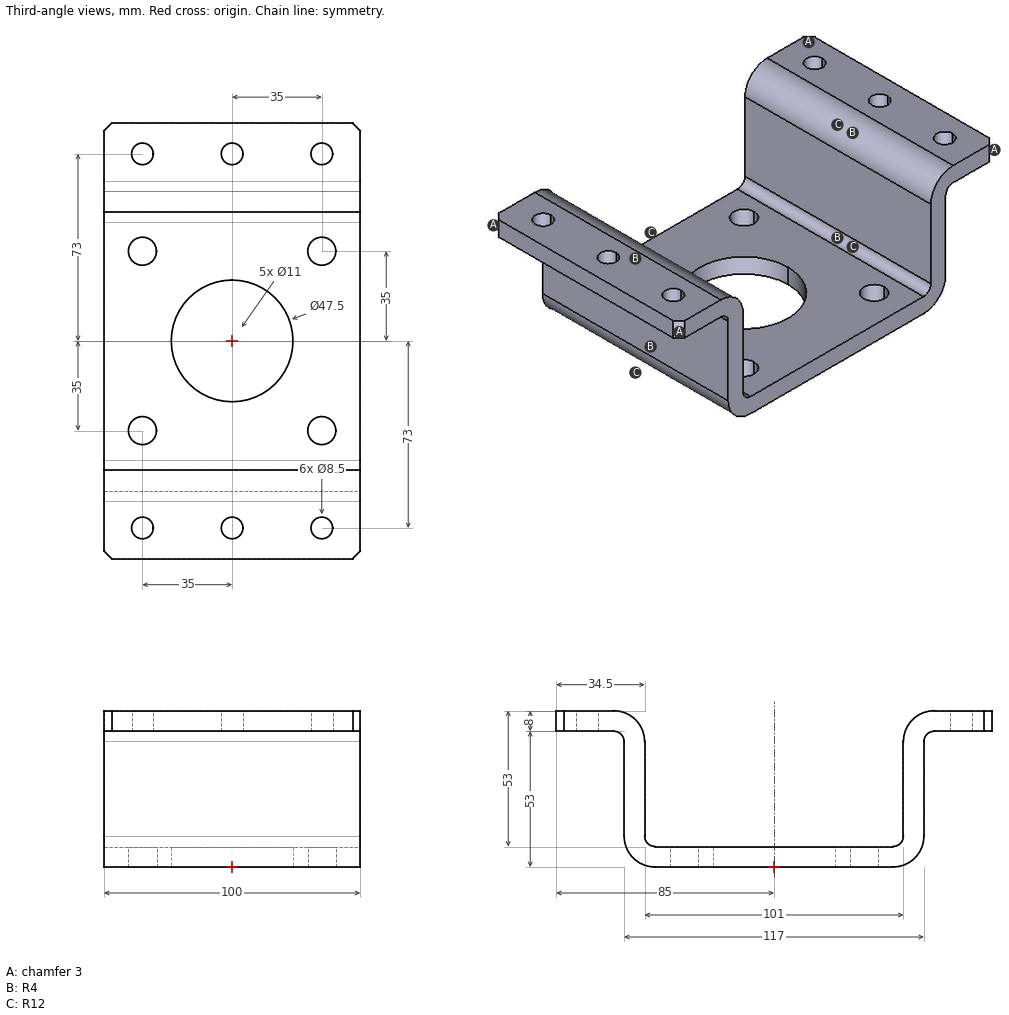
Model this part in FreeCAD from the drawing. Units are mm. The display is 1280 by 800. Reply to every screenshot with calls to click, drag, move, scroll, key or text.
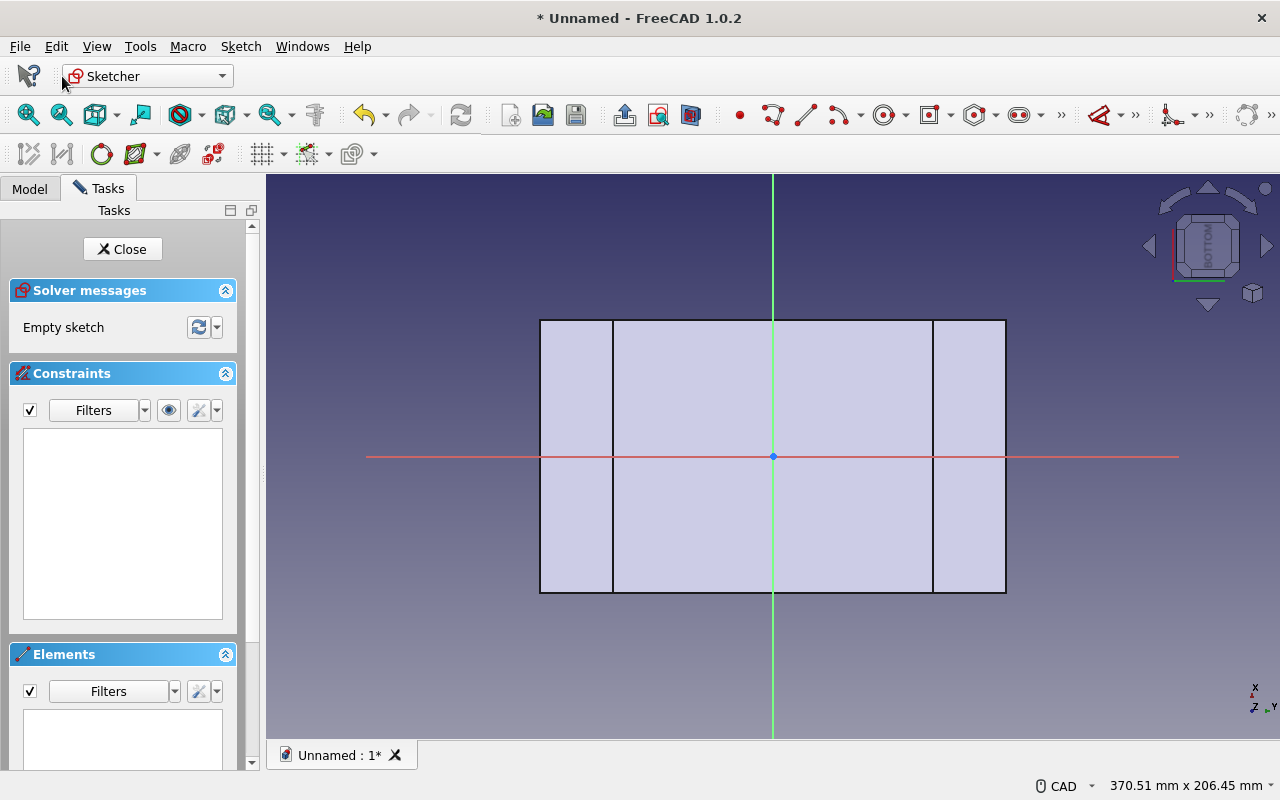
scroll(813, 456, up, 5)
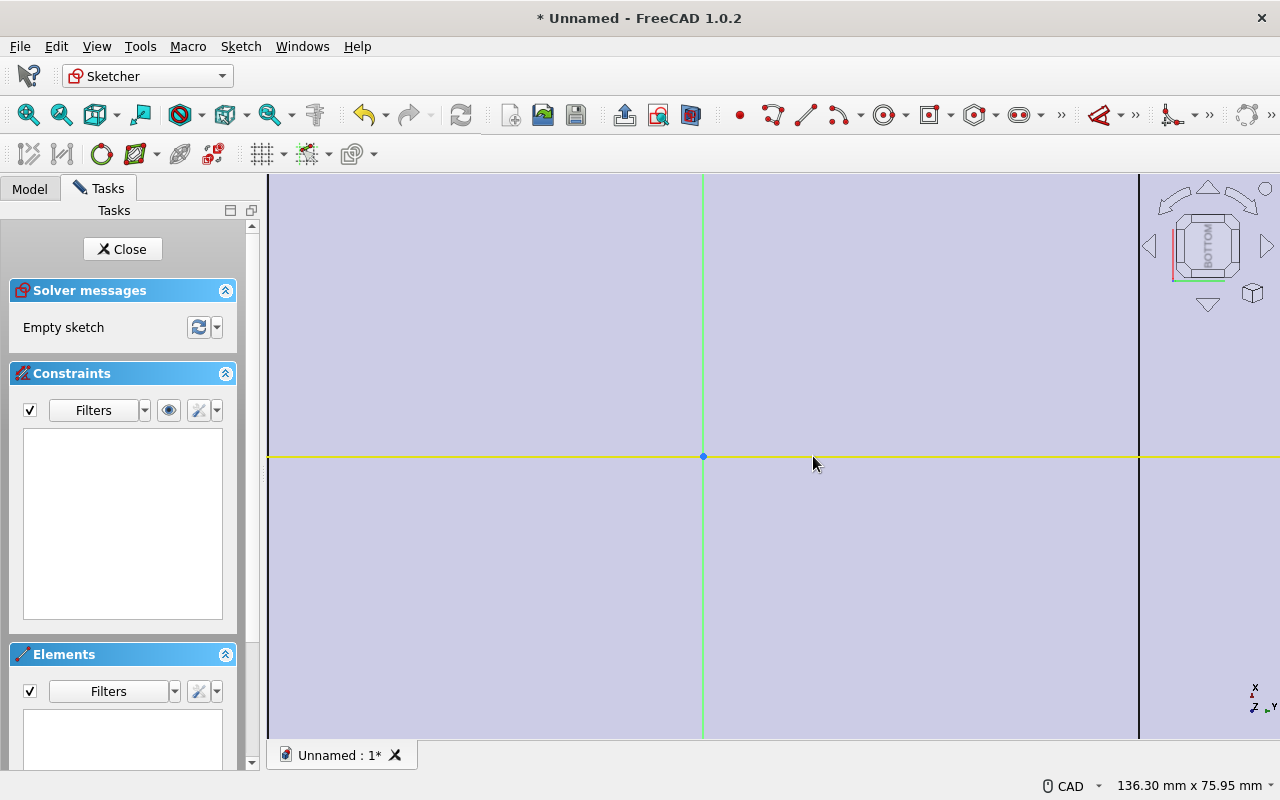
click(884, 116)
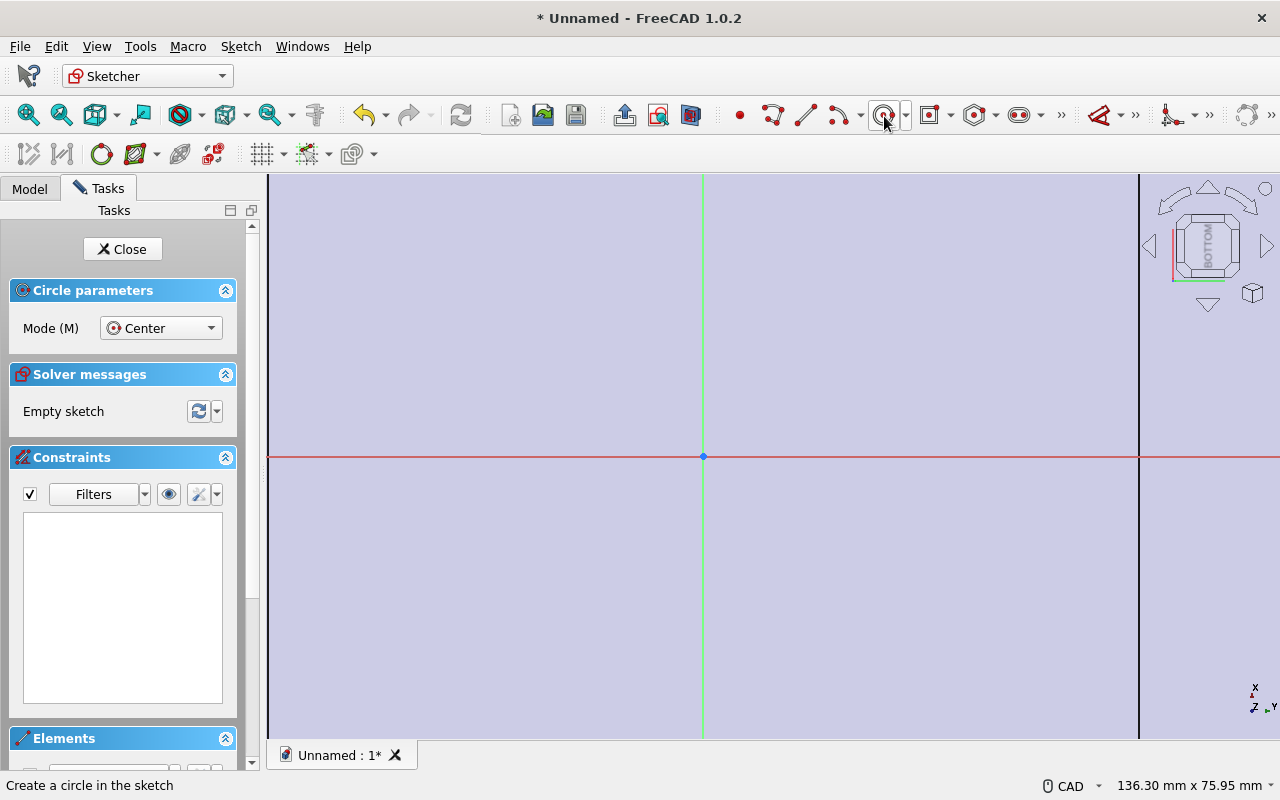
click(703, 456)
move(828, 332)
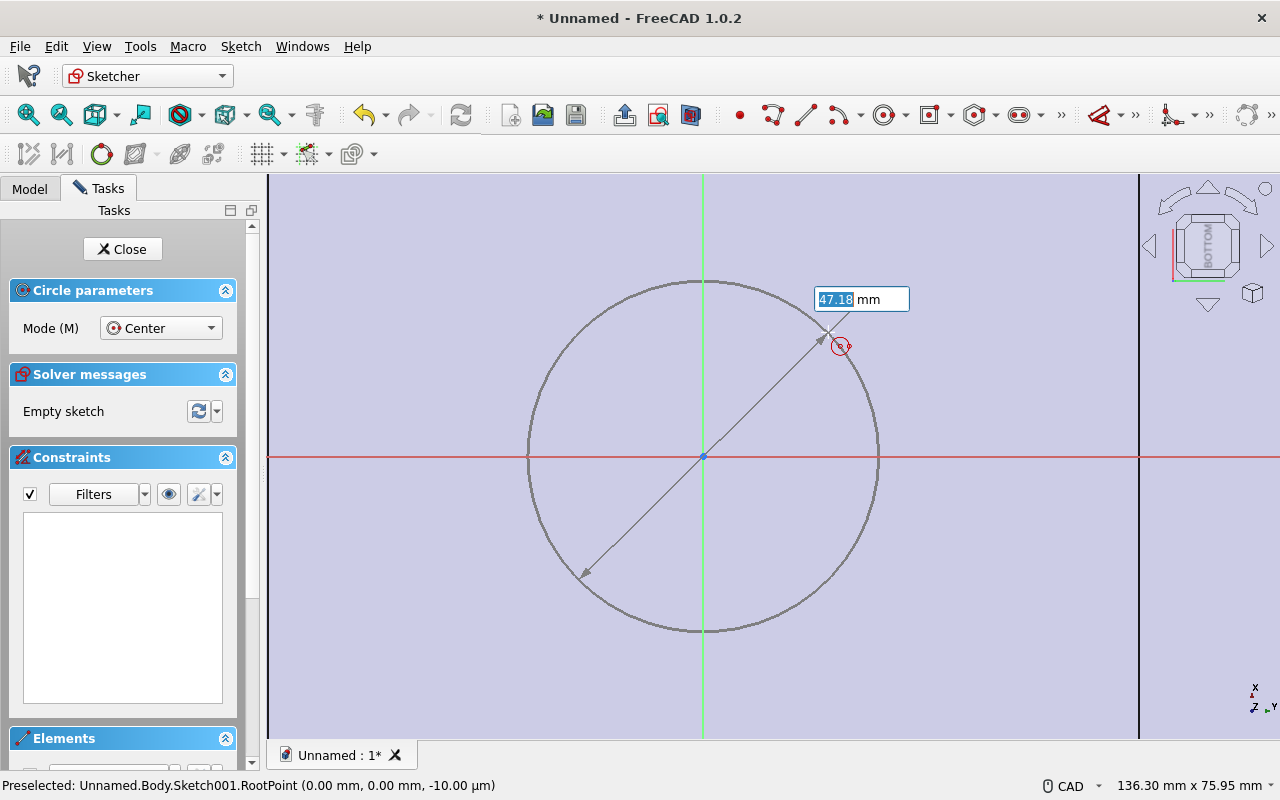
text(47.5)
key(Return)
key(Escape)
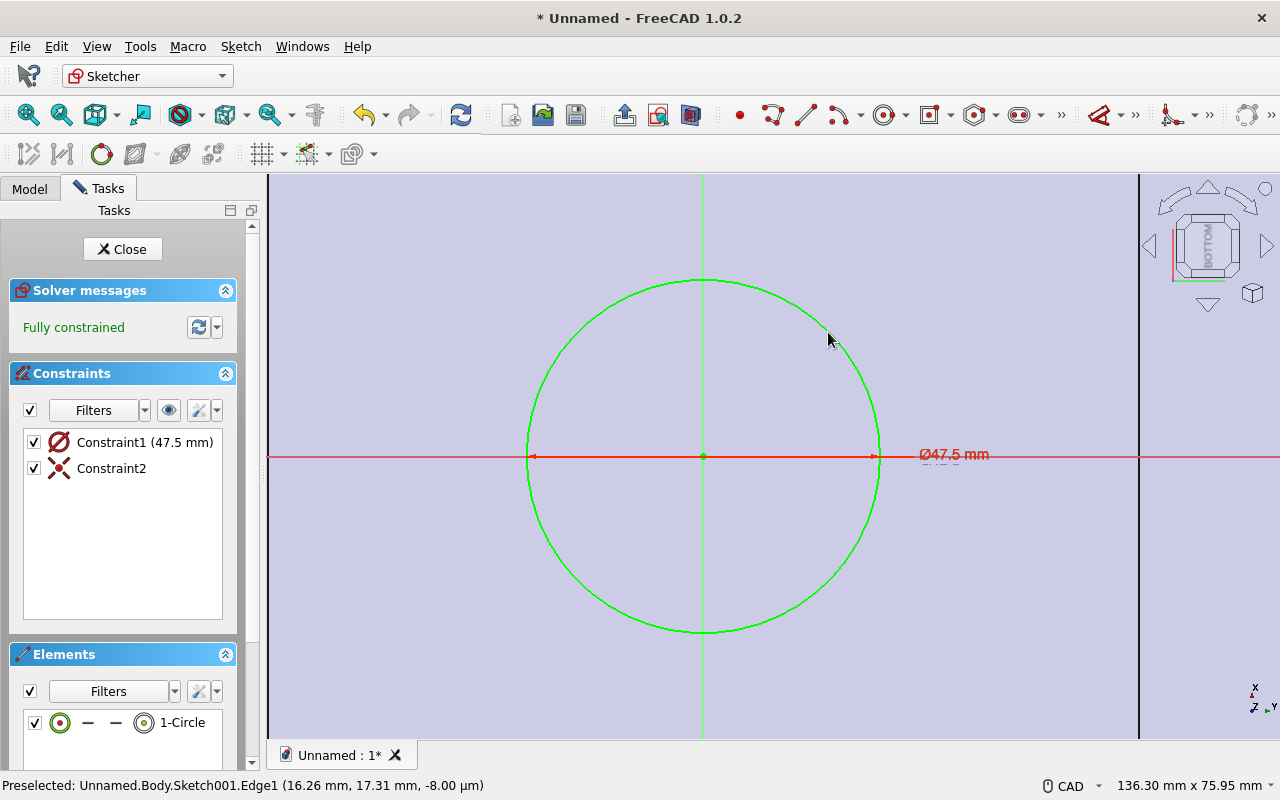
click(123, 249)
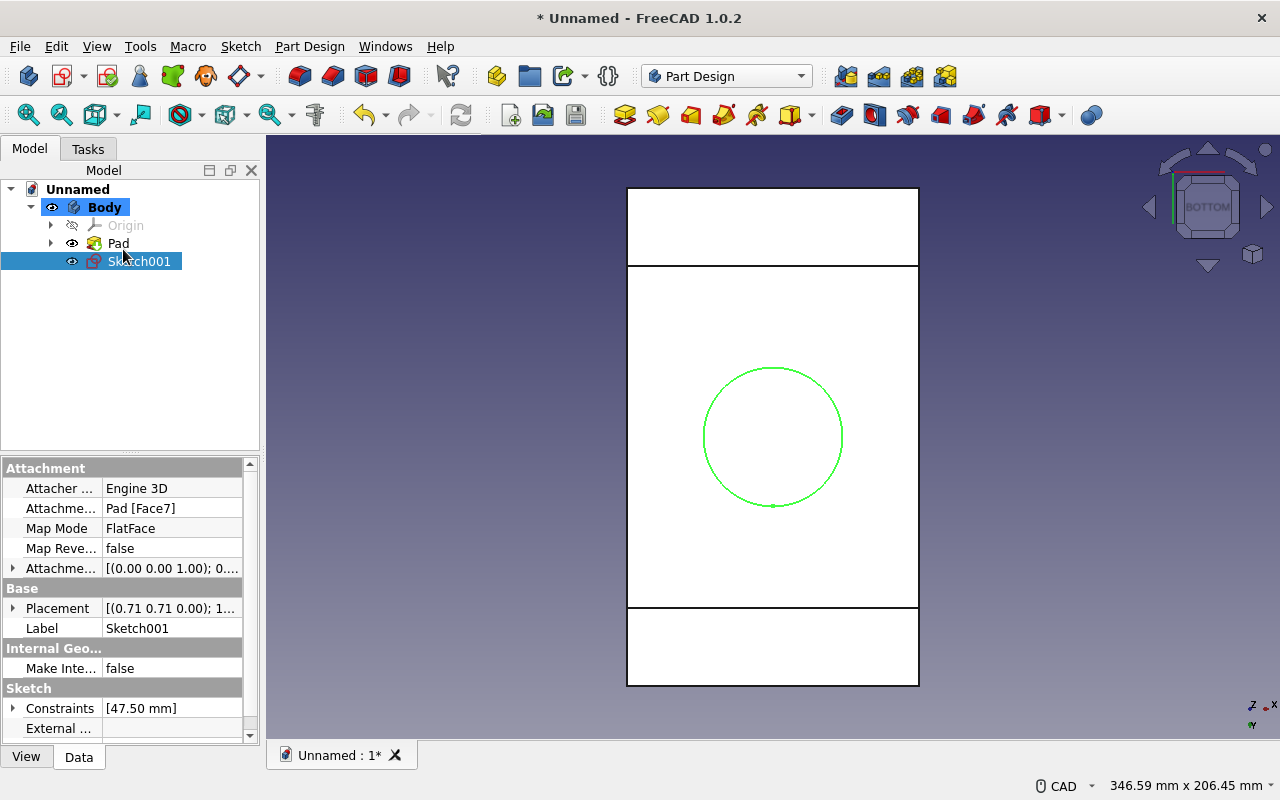
click(842, 116)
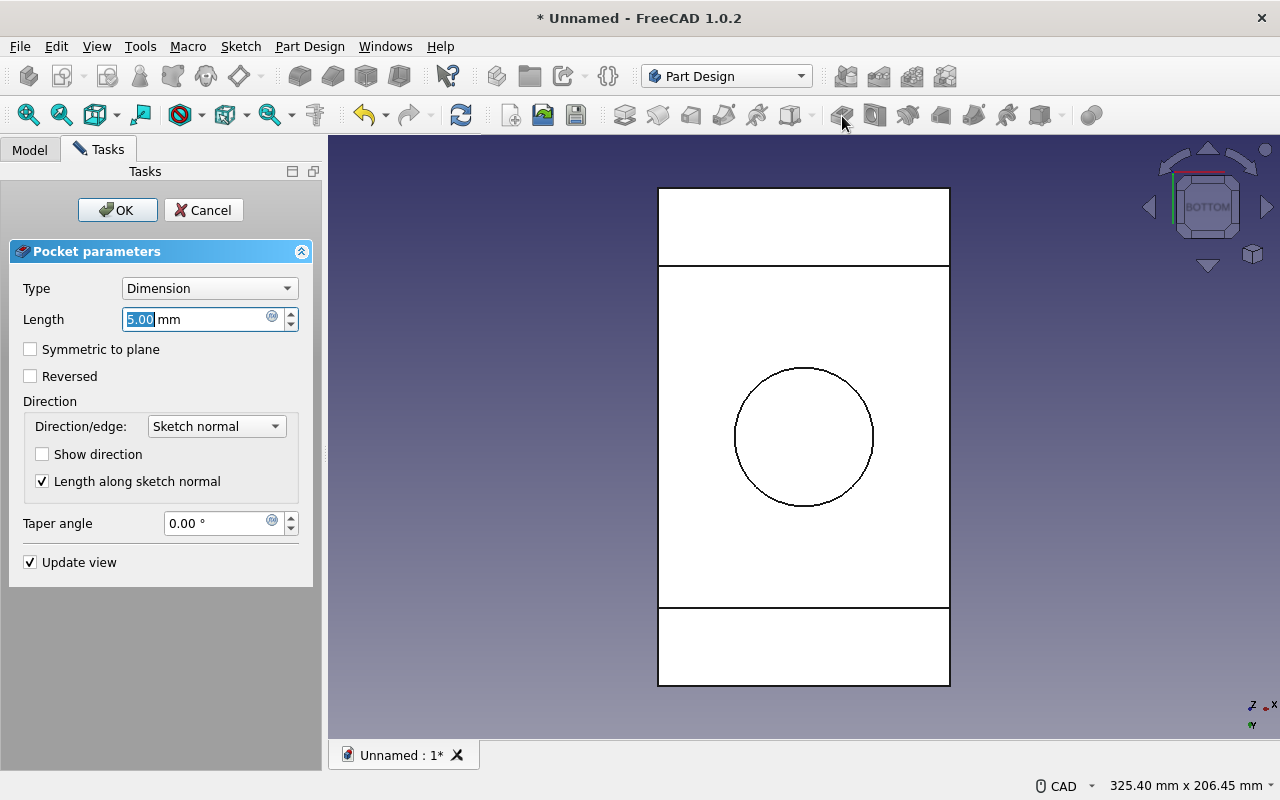
click(210, 288)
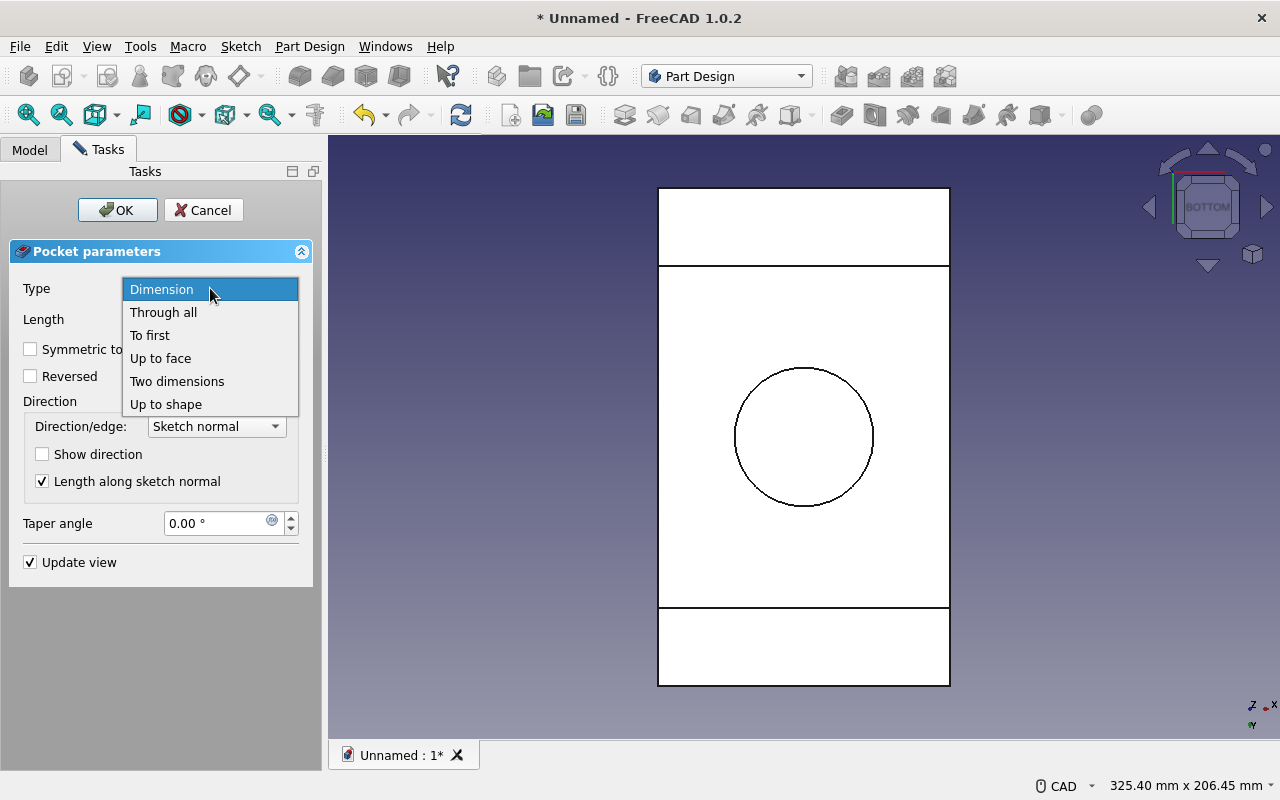
click(208, 312)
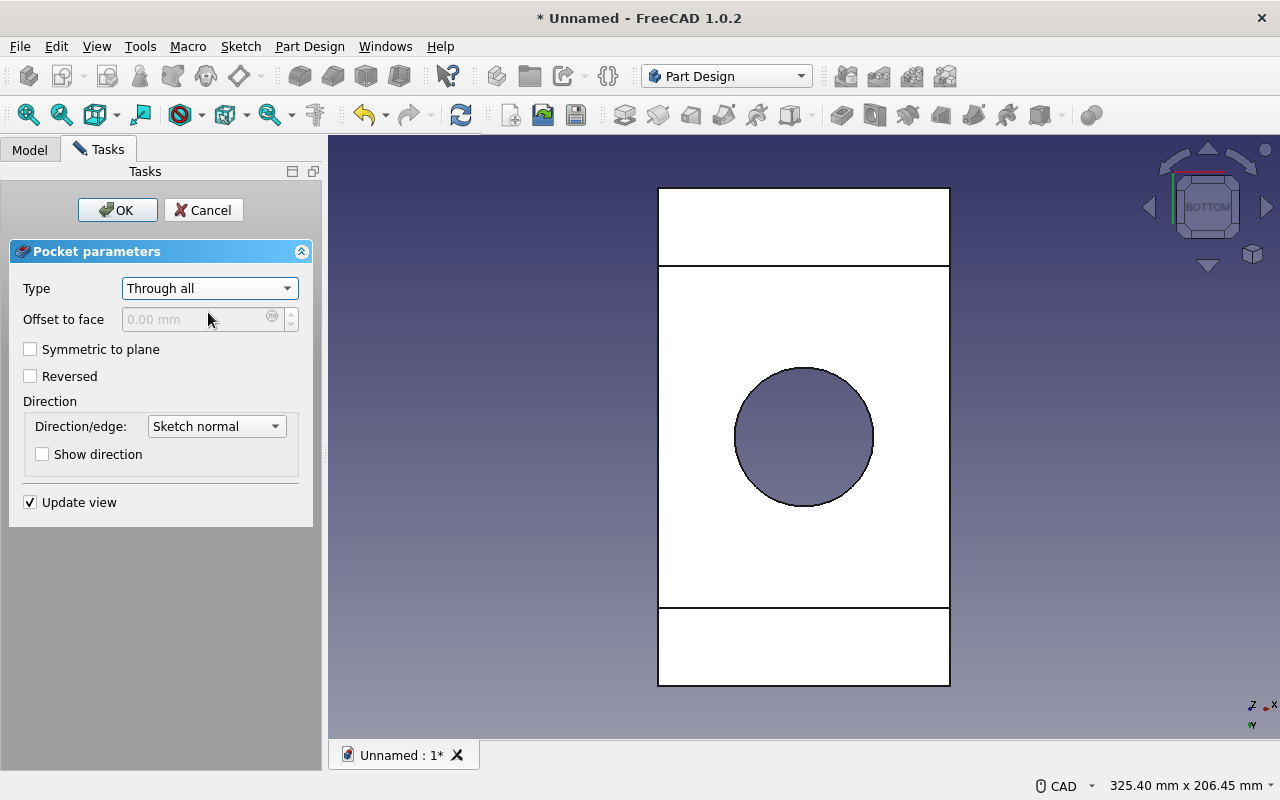
click(118, 210)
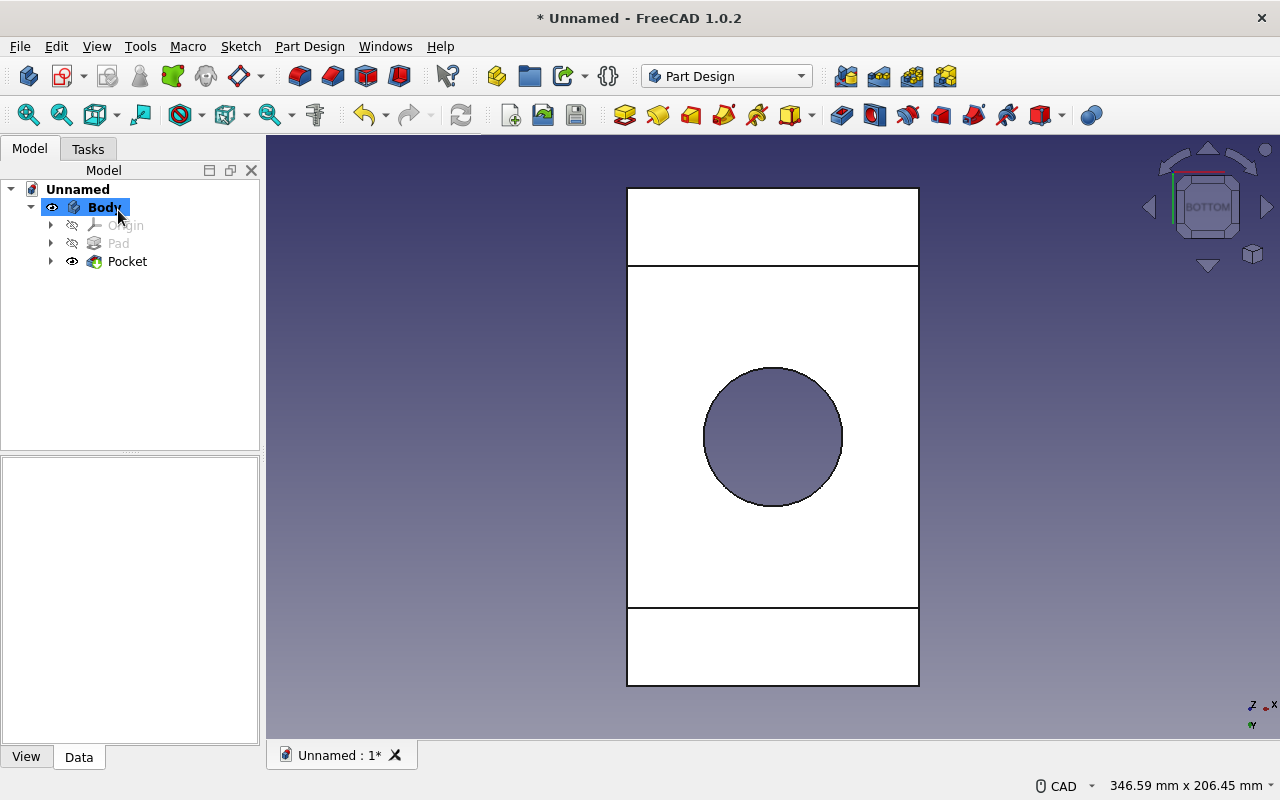
click(857, 338)